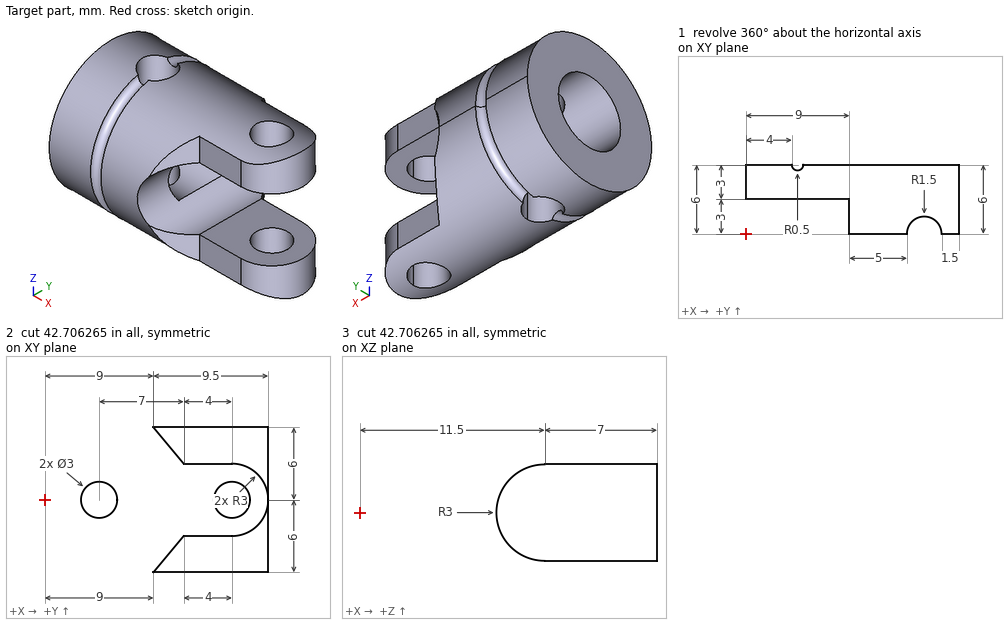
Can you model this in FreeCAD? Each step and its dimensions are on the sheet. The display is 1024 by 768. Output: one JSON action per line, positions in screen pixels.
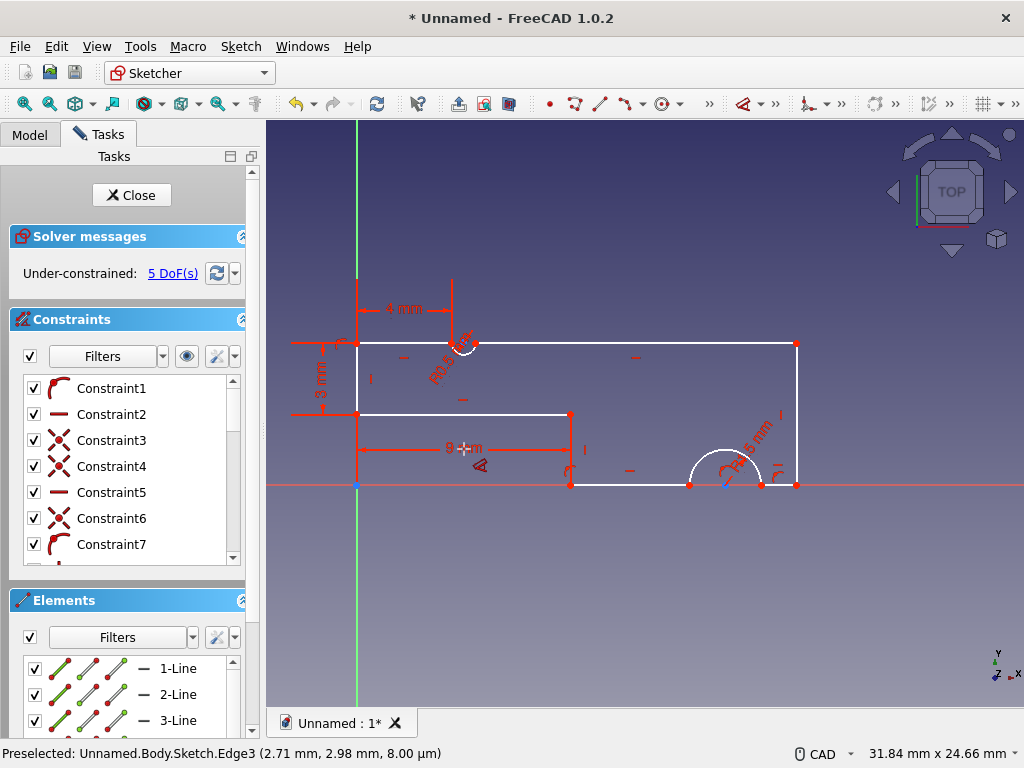
{"action": "left_click", "coordinate": [571, 436]}
{"action": "left_click", "coordinate": [537, 450]}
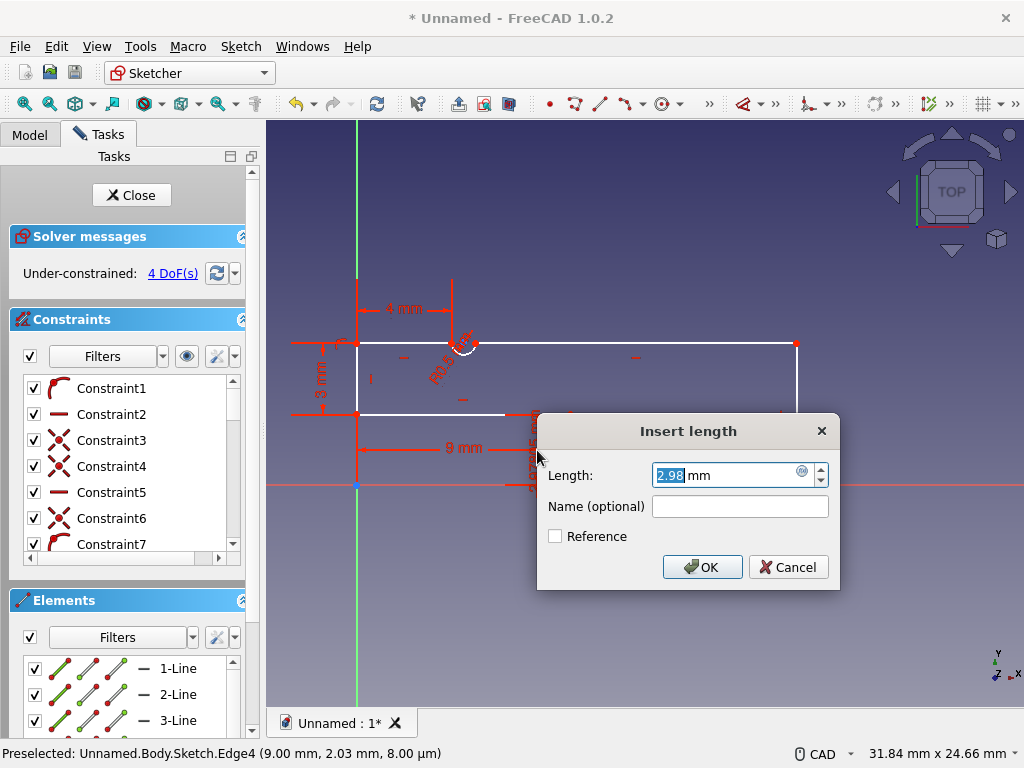
{"action": "type", "text": "3"}
{"action": "key", "text": "Return"}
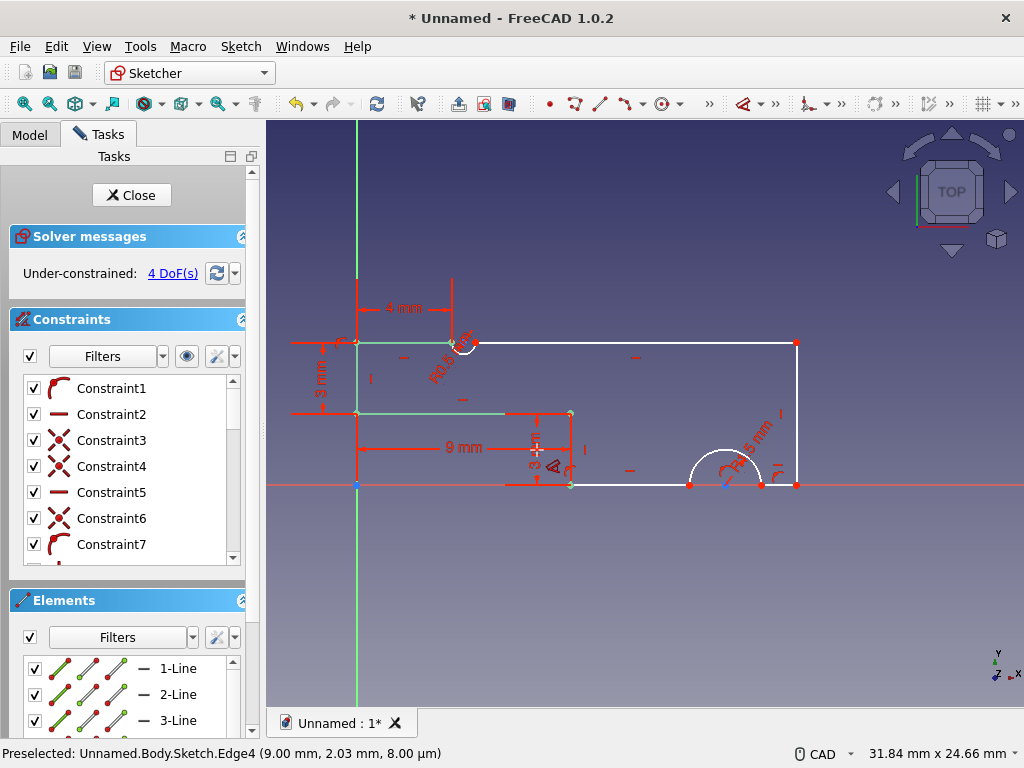
{"action": "left_click", "coordinate": [606, 485]}
{"action": "left_click", "coordinate": [630, 519]}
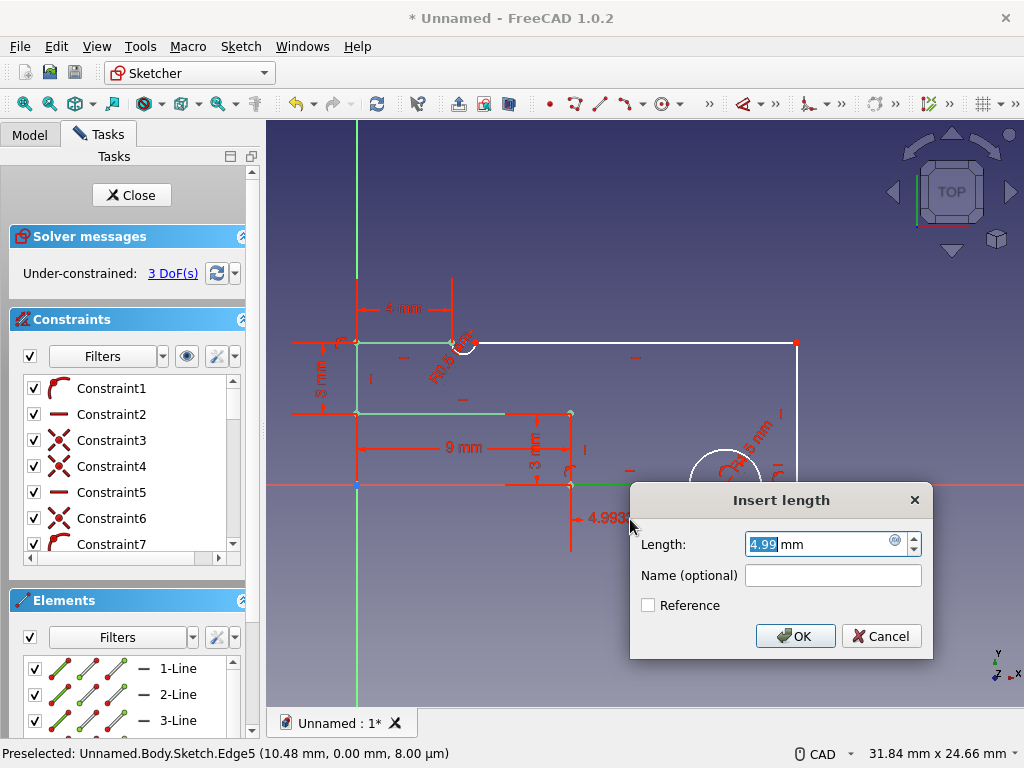
{"action": "type", "text": "5"}
{"action": "key", "text": "Return"}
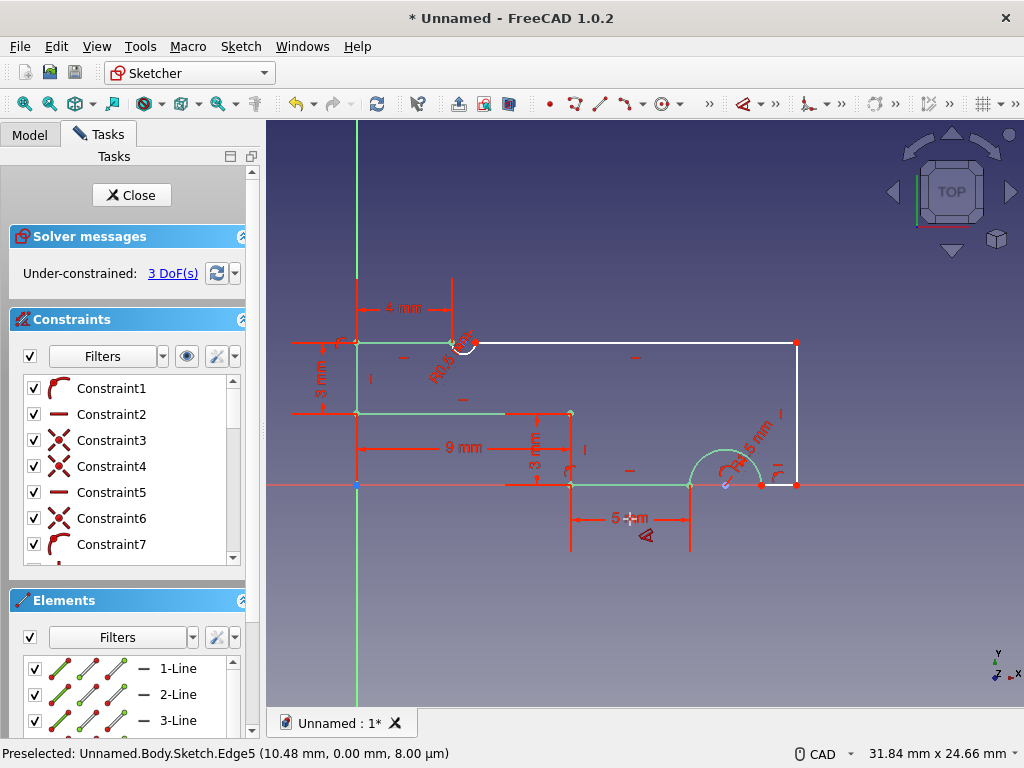
{"action": "left_click", "coordinate": [797, 443]}
{"action": "left_click", "coordinate": [831, 414]}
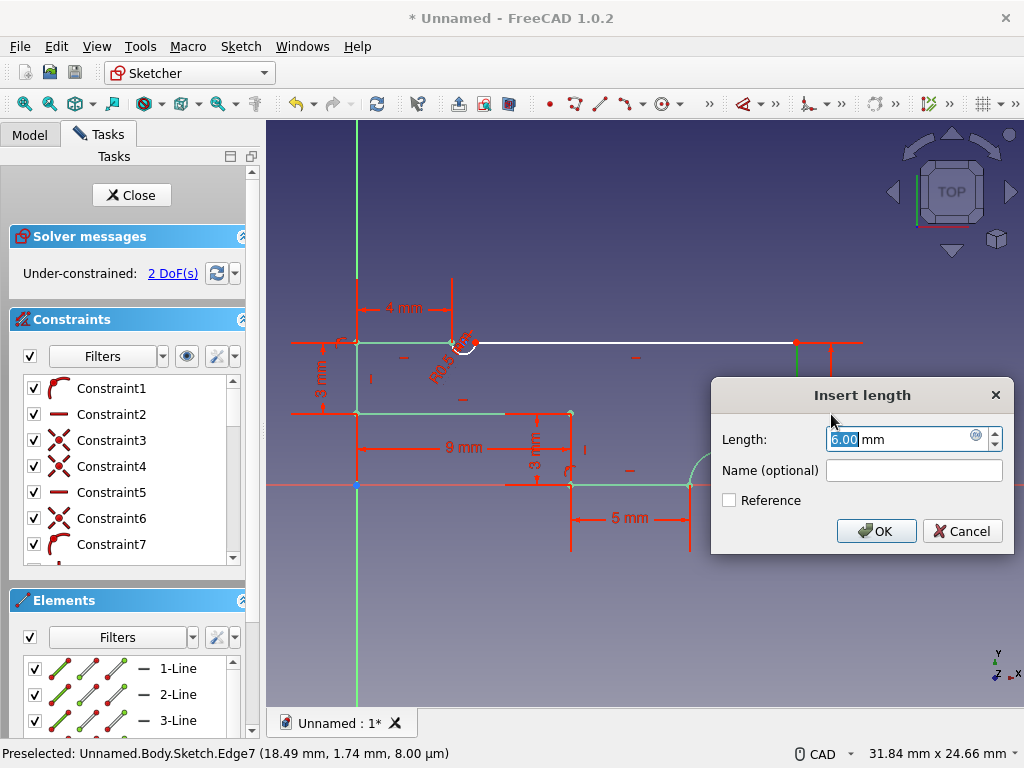
{"action": "type", "text": "6"}
{"action": "key", "text": "Return"}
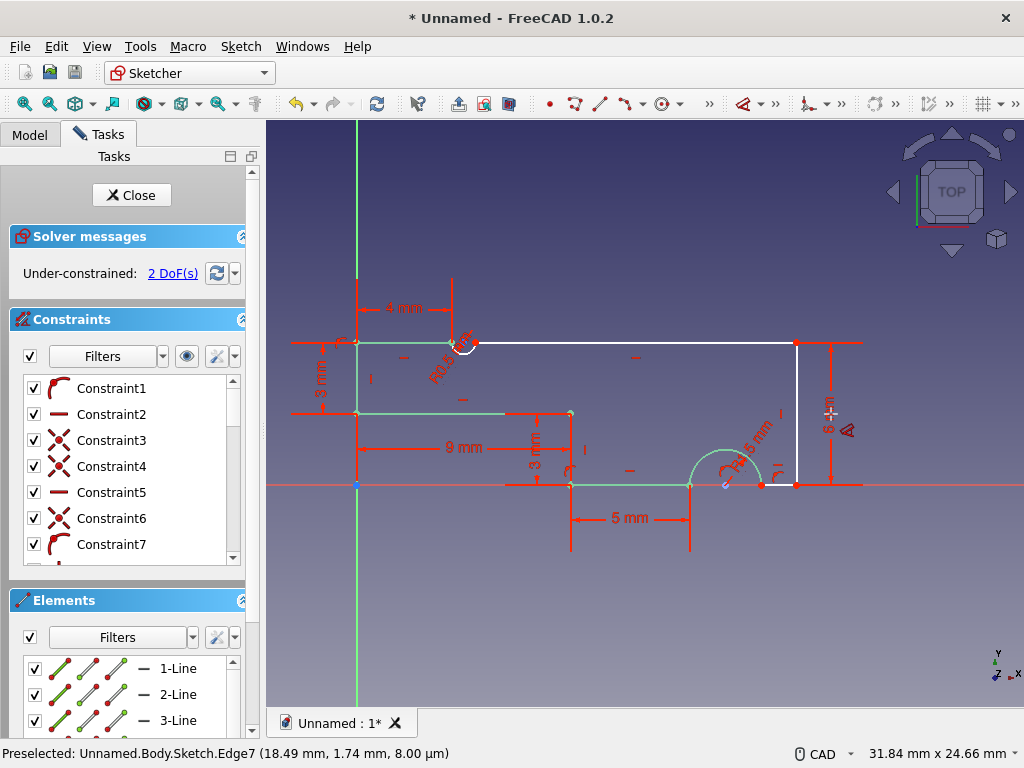
{"action": "left_click", "coordinate": [464, 342]}
{"action": "left_click", "coordinate": [323, 414]}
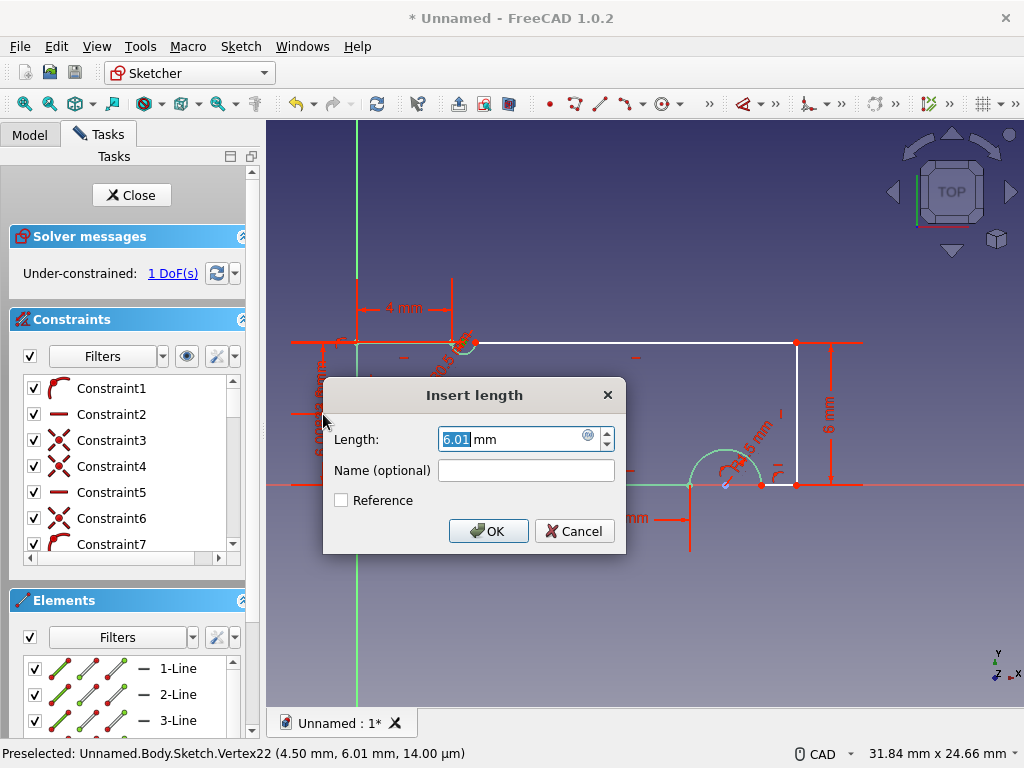
{"action": "type", "text": "6"}
{"action": "key", "text": "Return"}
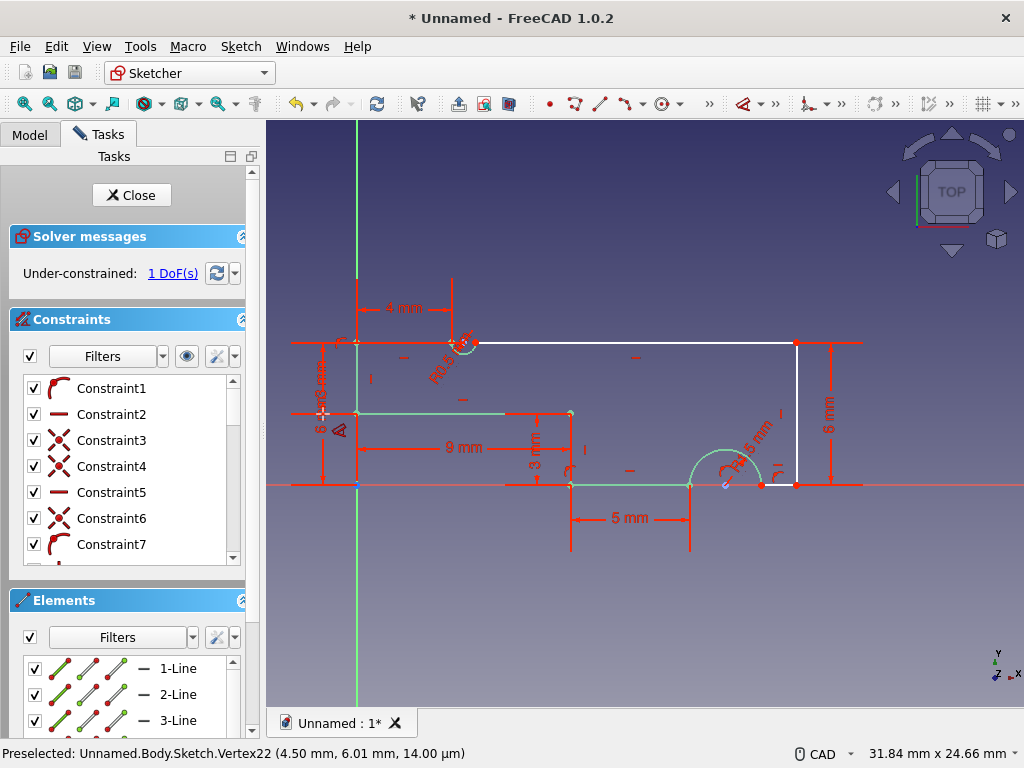
{"action": "scroll", "coordinate": [772, 485], "scroll_direction": "up", "scroll_amount": 2}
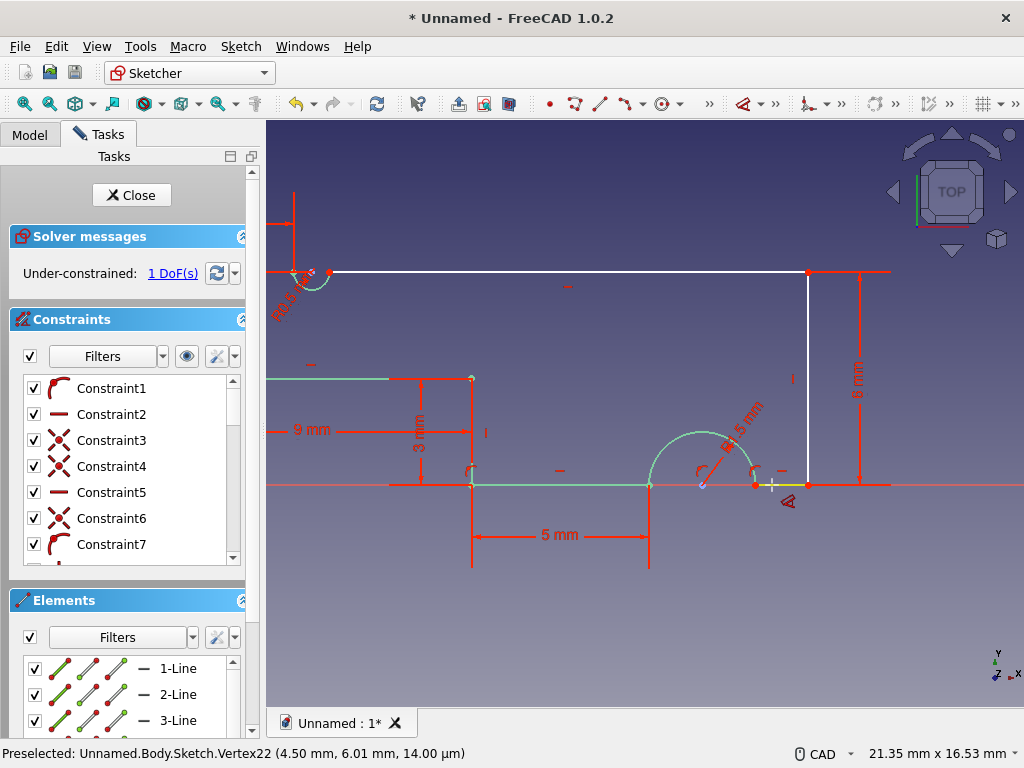
{"action": "left_click", "coordinate": [771, 485]}
{"action": "left_click", "coordinate": [782, 519]}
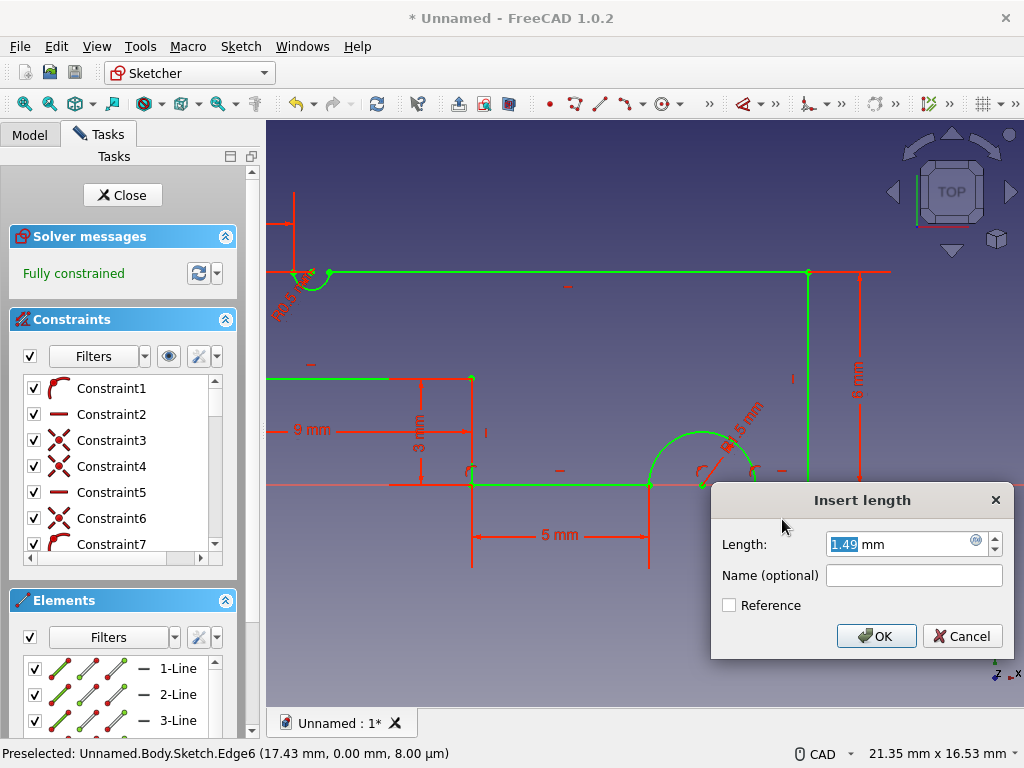
{"action": "type", "text": "1.5"}
{"action": "key", "text": "Return"}
{"action": "key", "text": "Escape"}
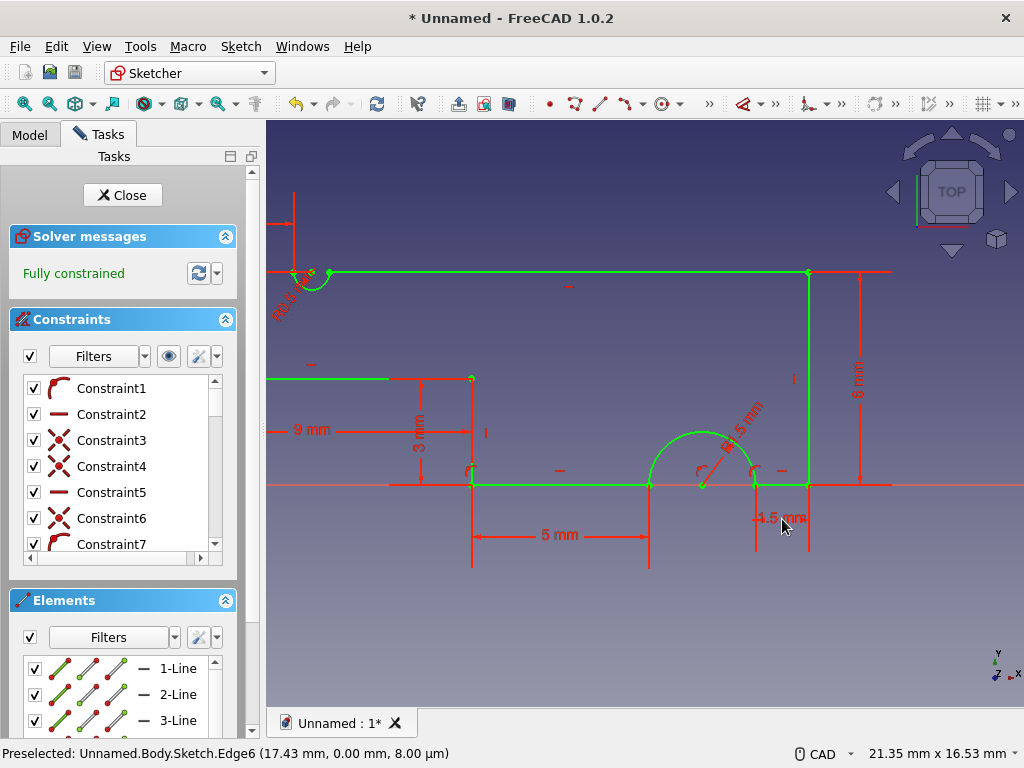
{"action": "left_click", "coordinate": [123, 195]}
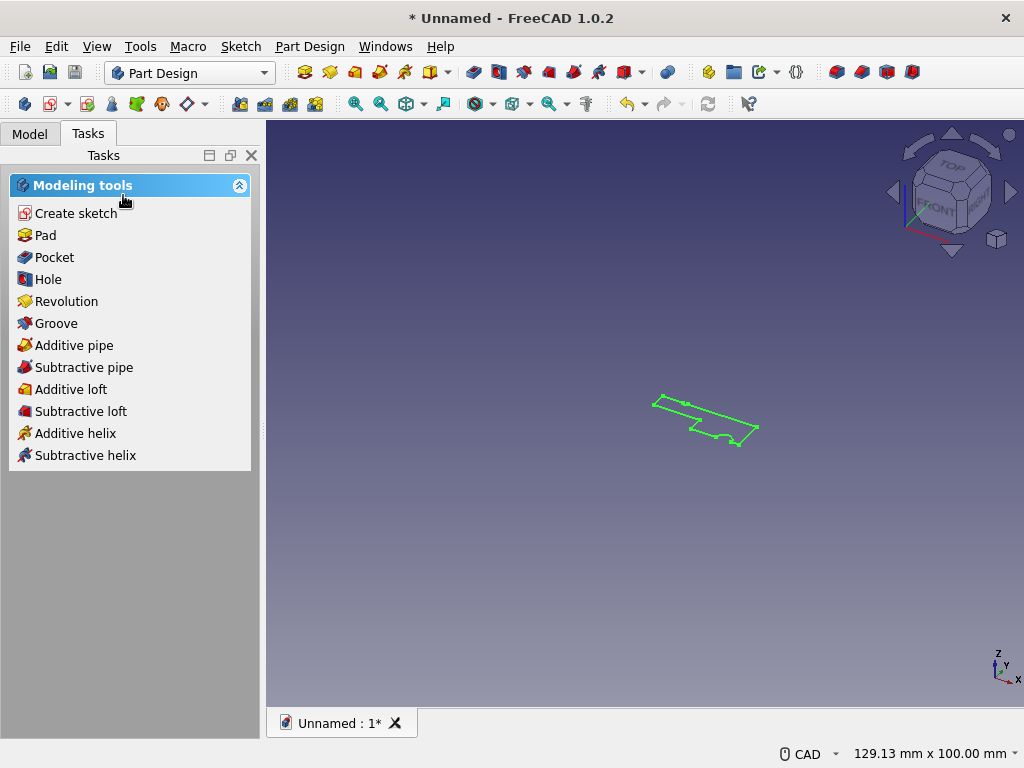
{"action": "left_click", "coordinate": [330, 72]}